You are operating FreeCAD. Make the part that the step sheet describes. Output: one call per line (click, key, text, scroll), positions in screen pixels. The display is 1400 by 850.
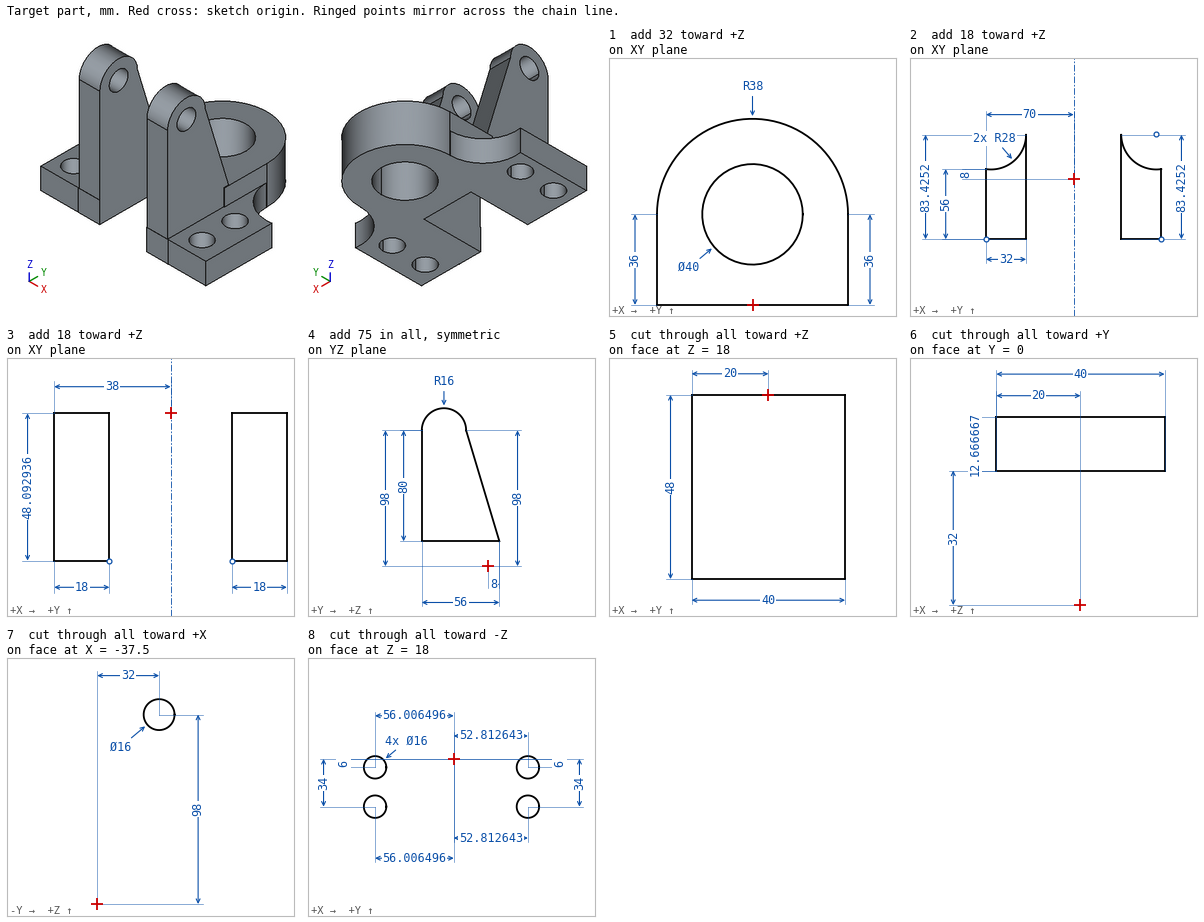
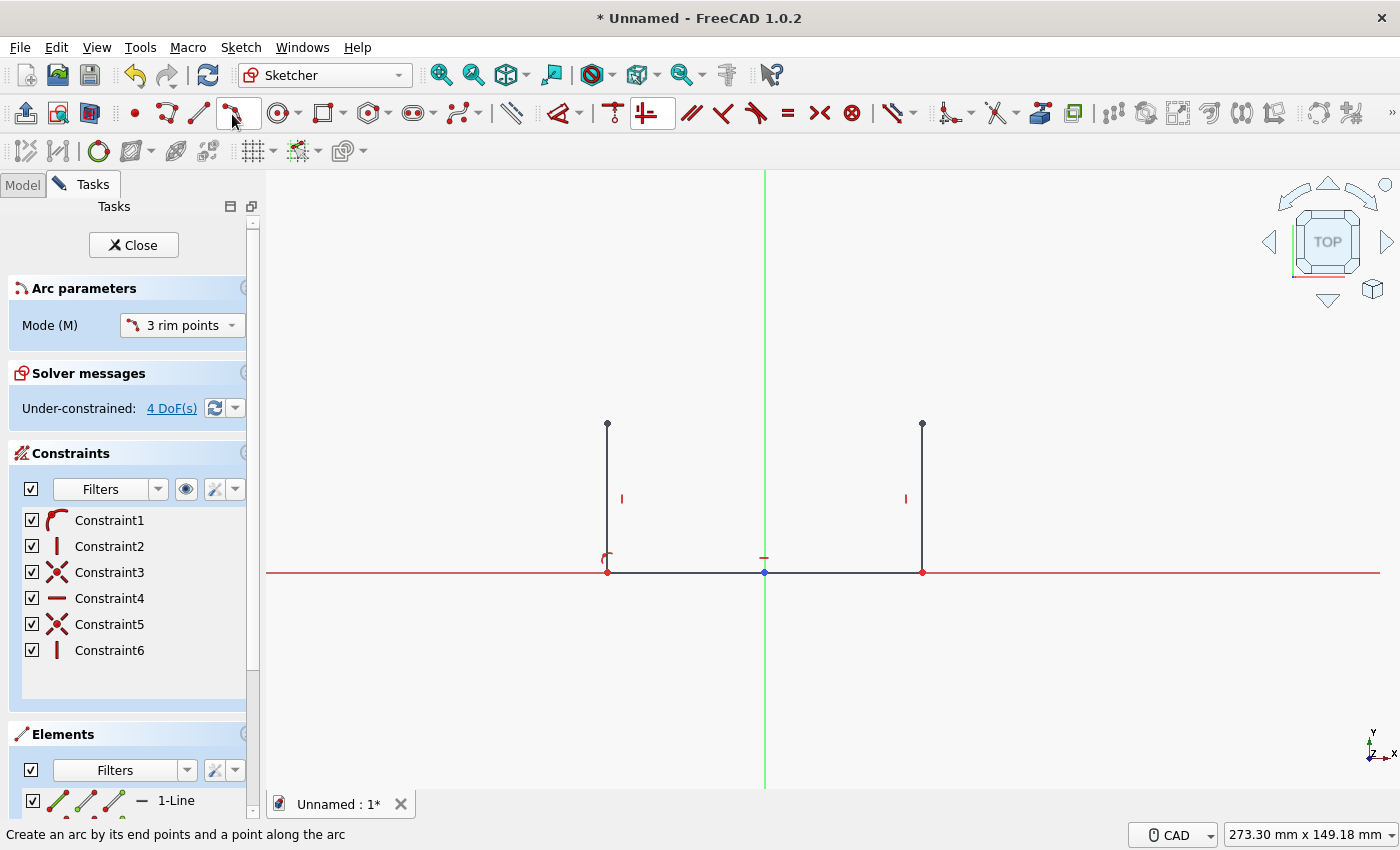
click(922, 424)
click(607, 424)
click(813, 273)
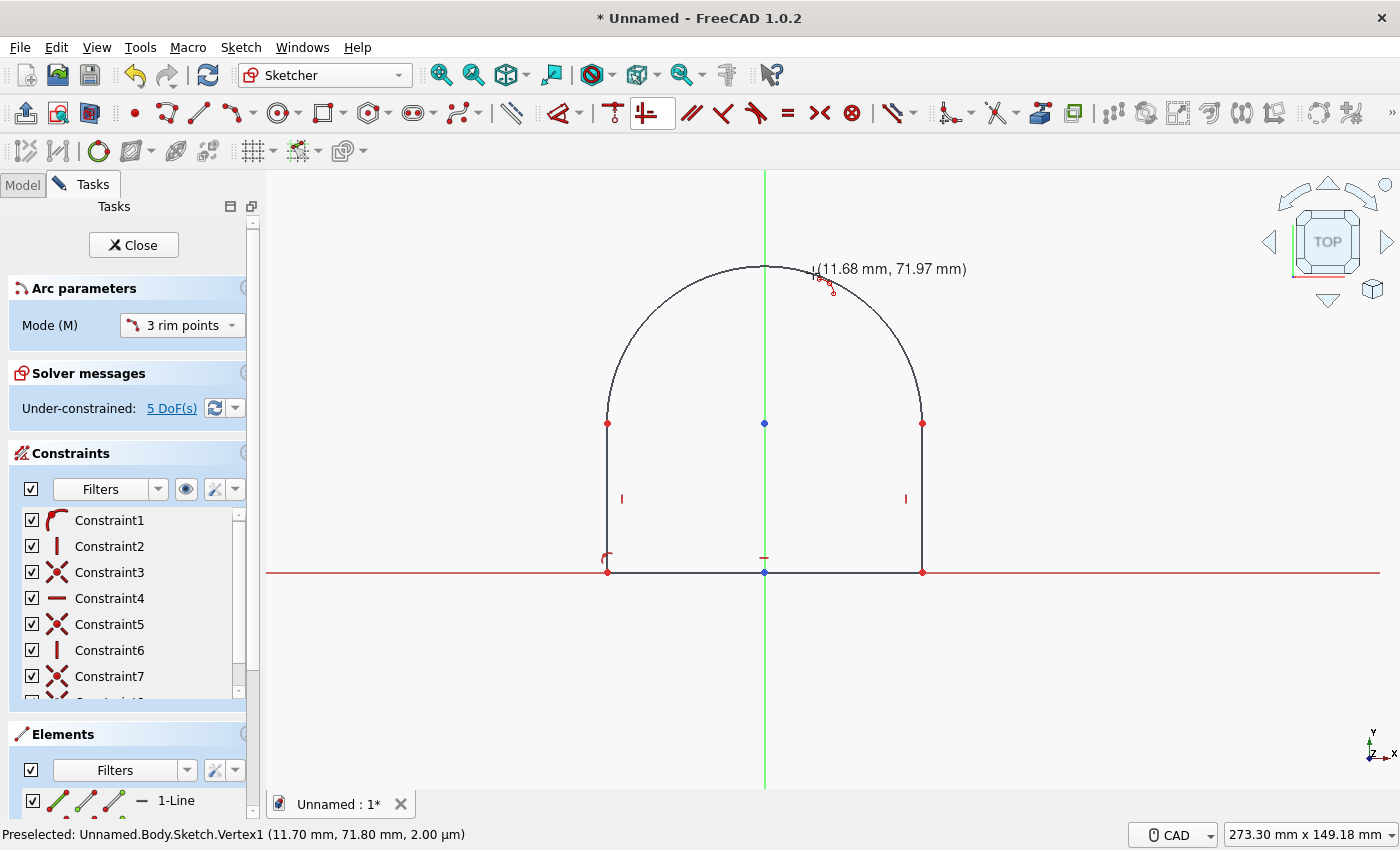
click(278, 114)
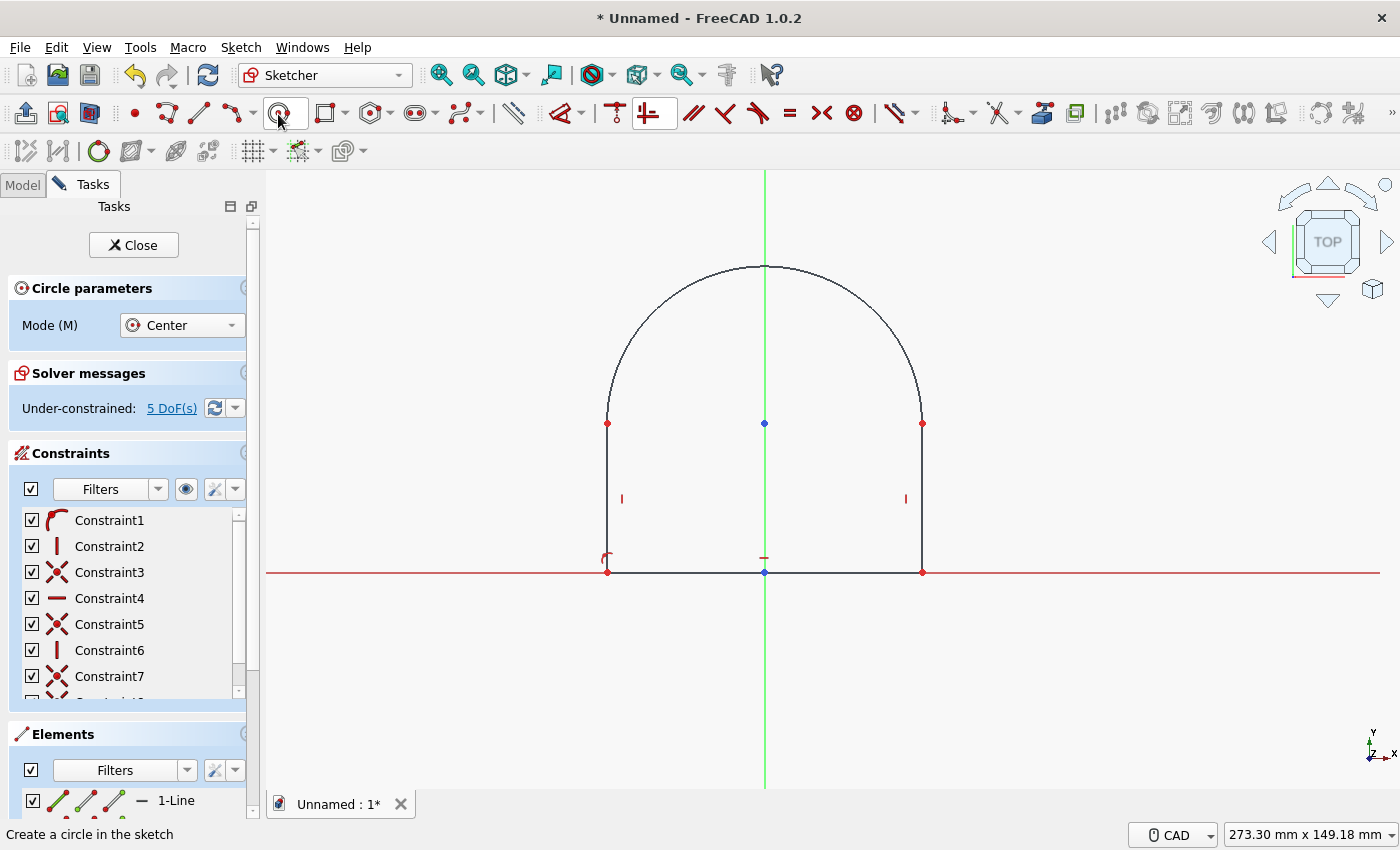
click(765, 423)
click(823, 365)
key(Escape)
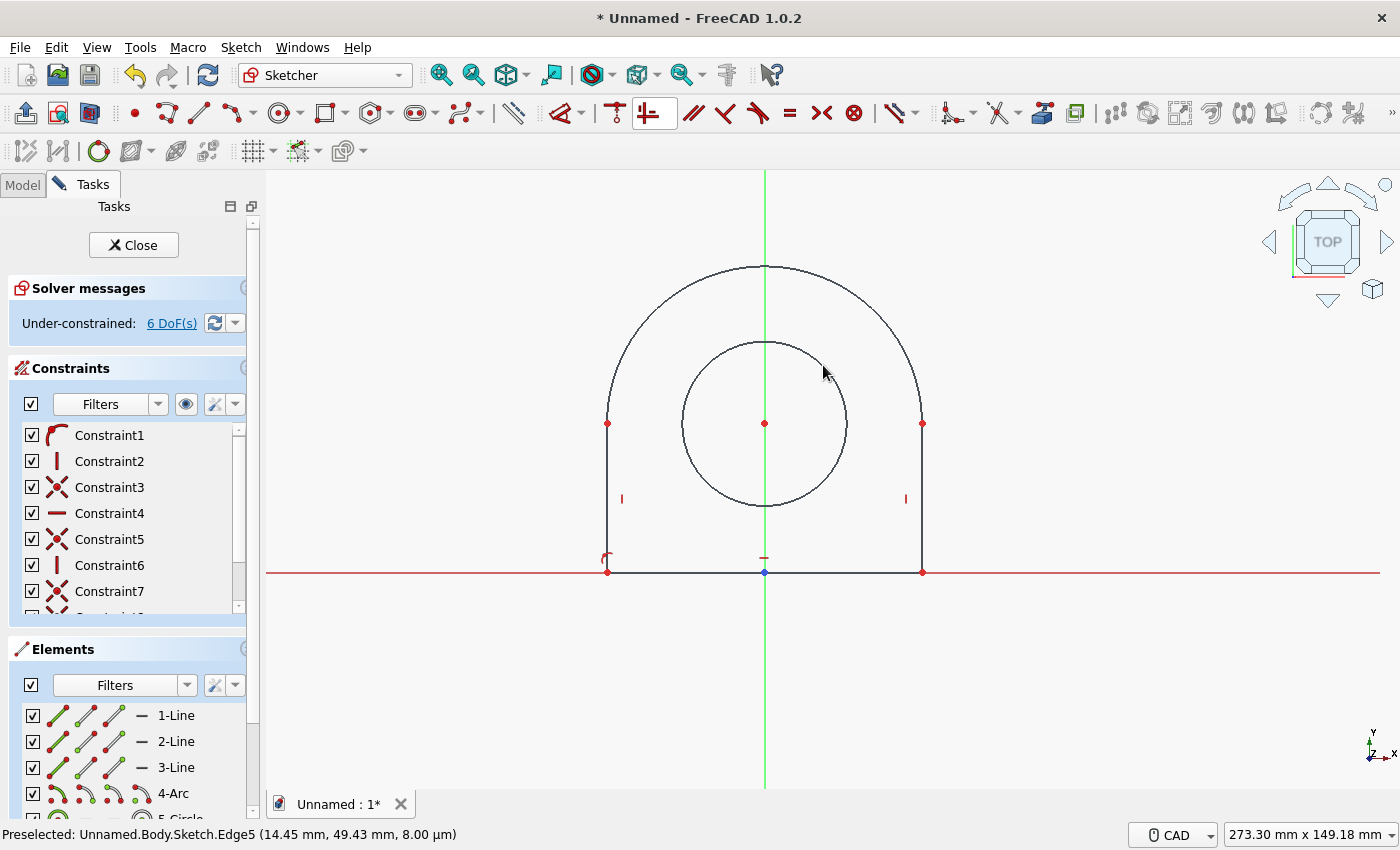
click(607, 469)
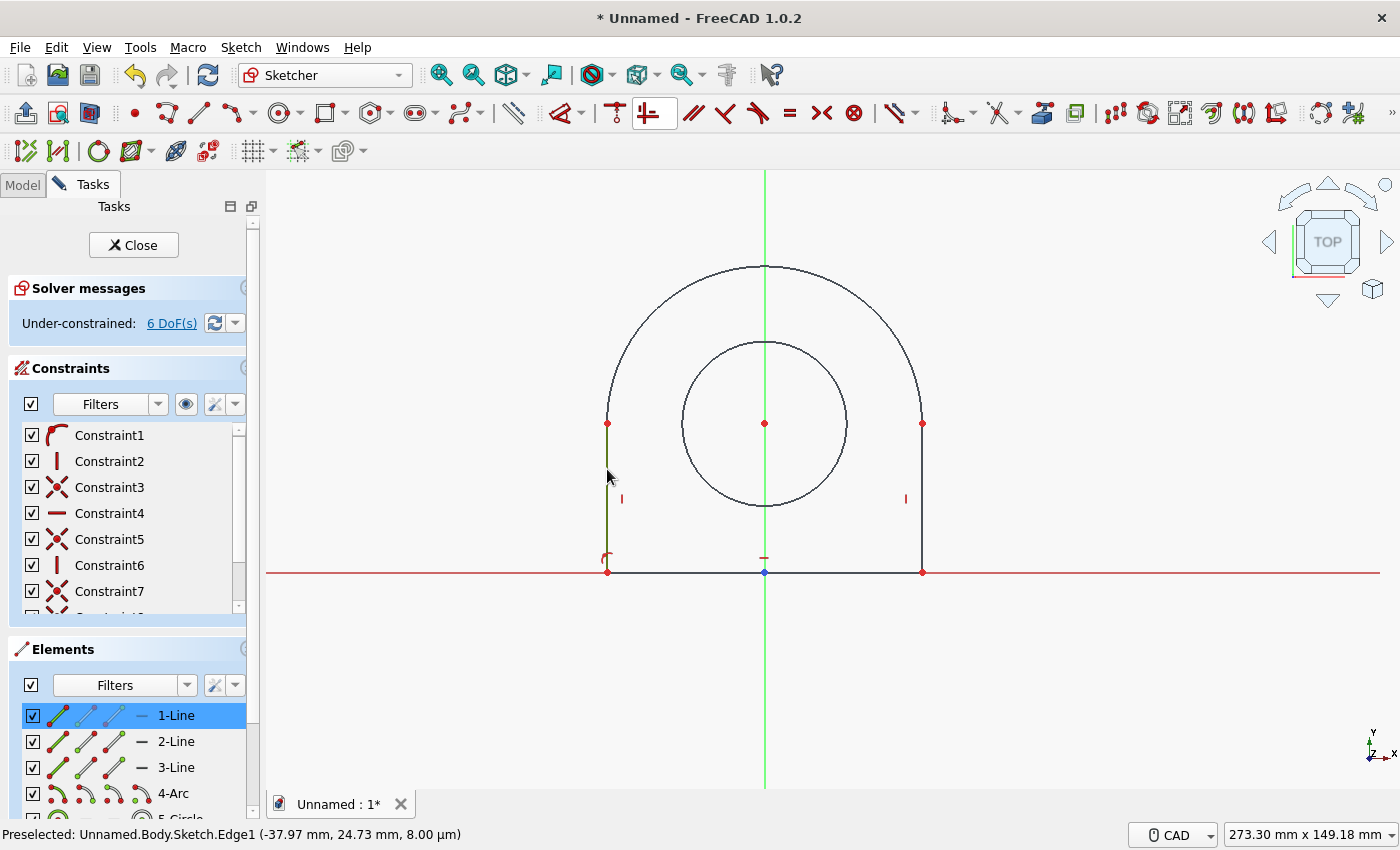
click(857, 296)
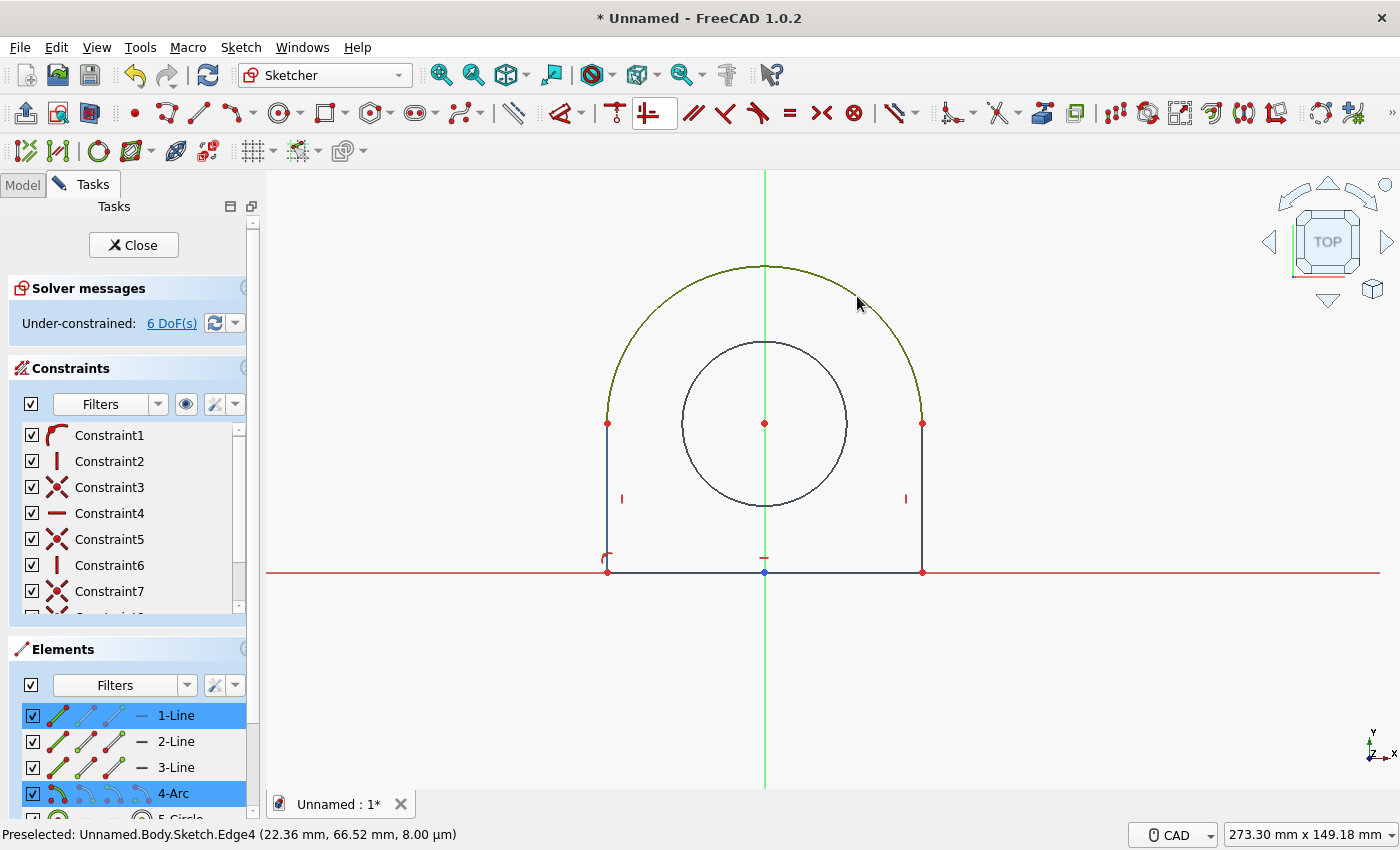
click(758, 114)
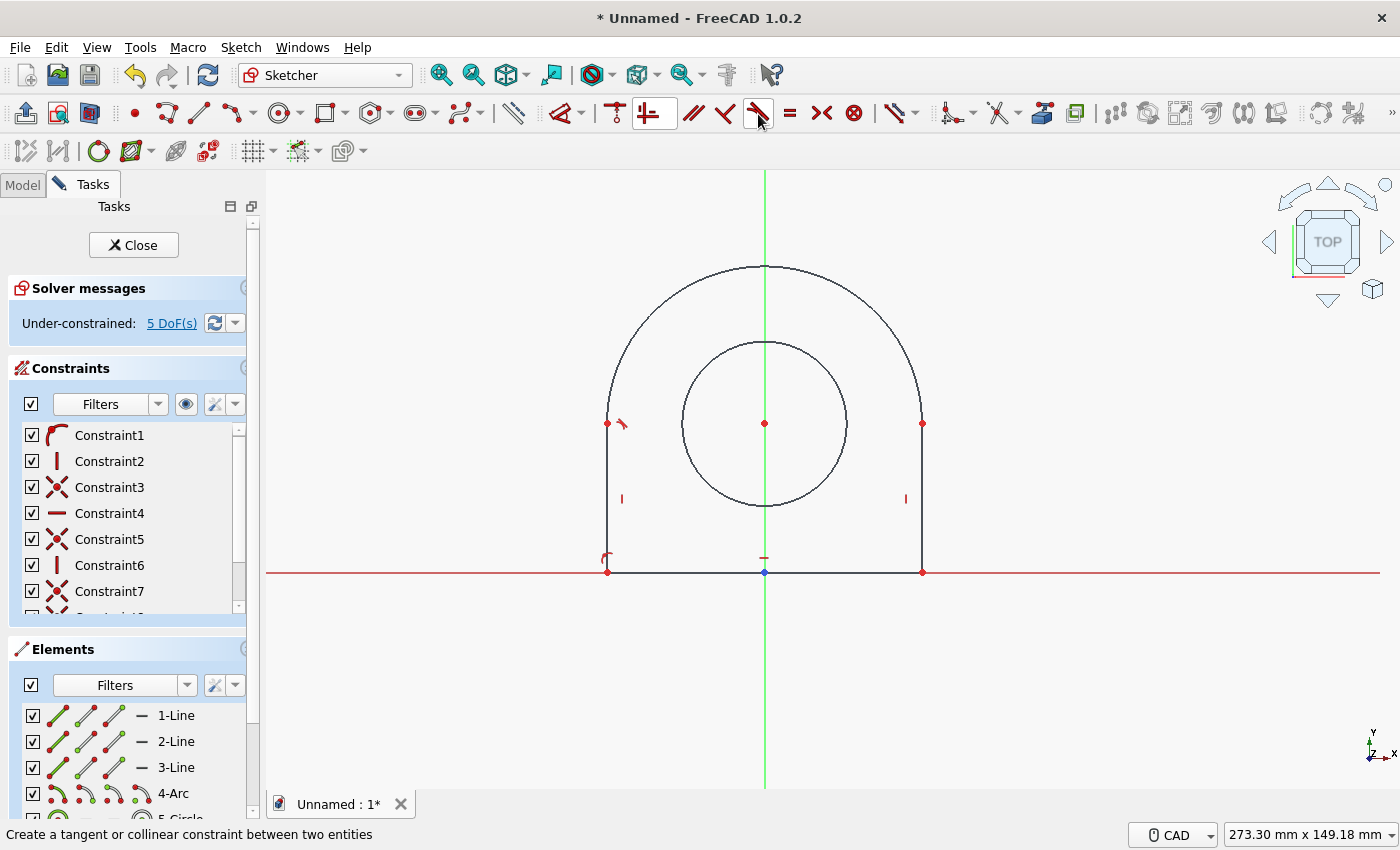
click(765, 424)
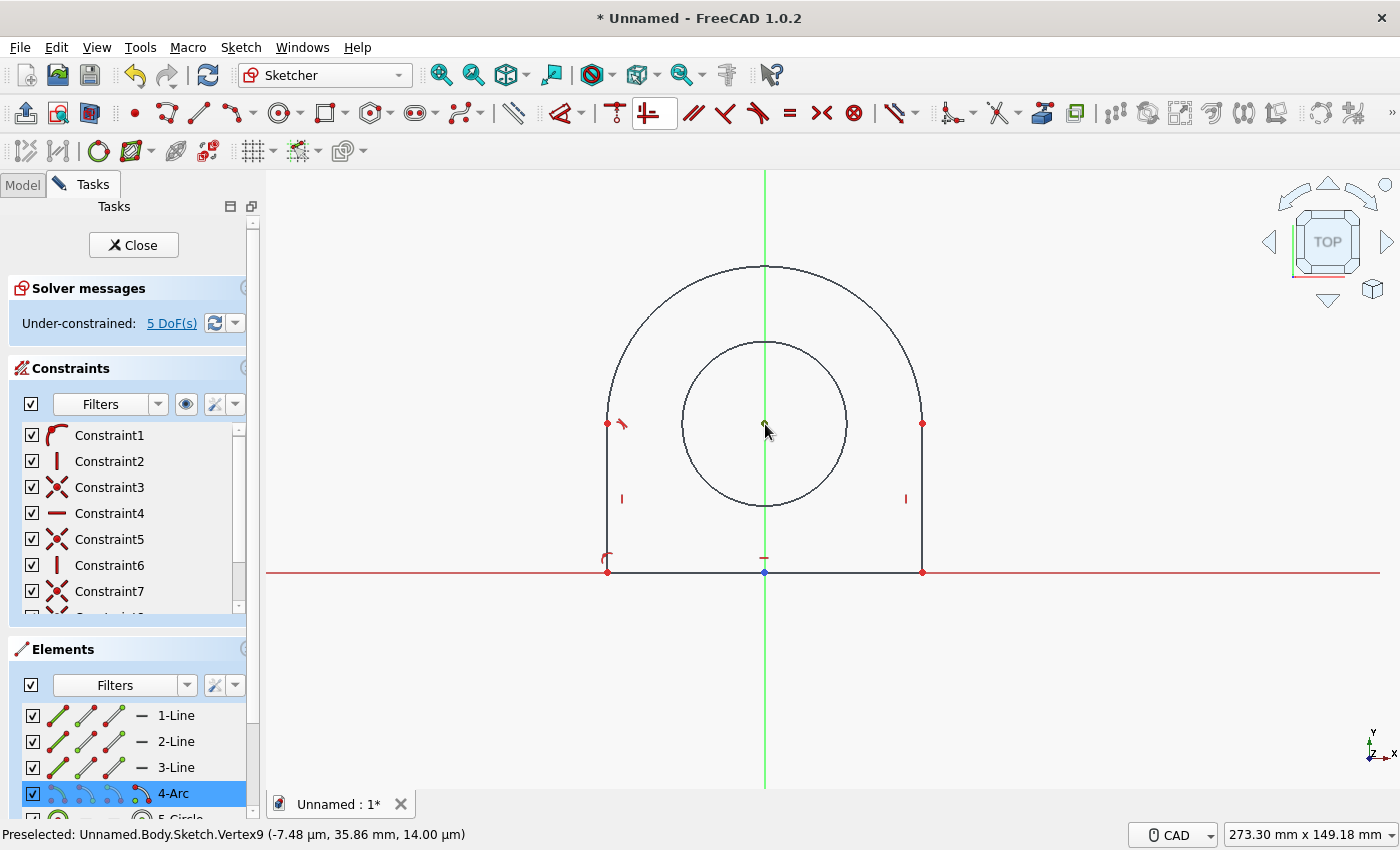
click(765, 721)